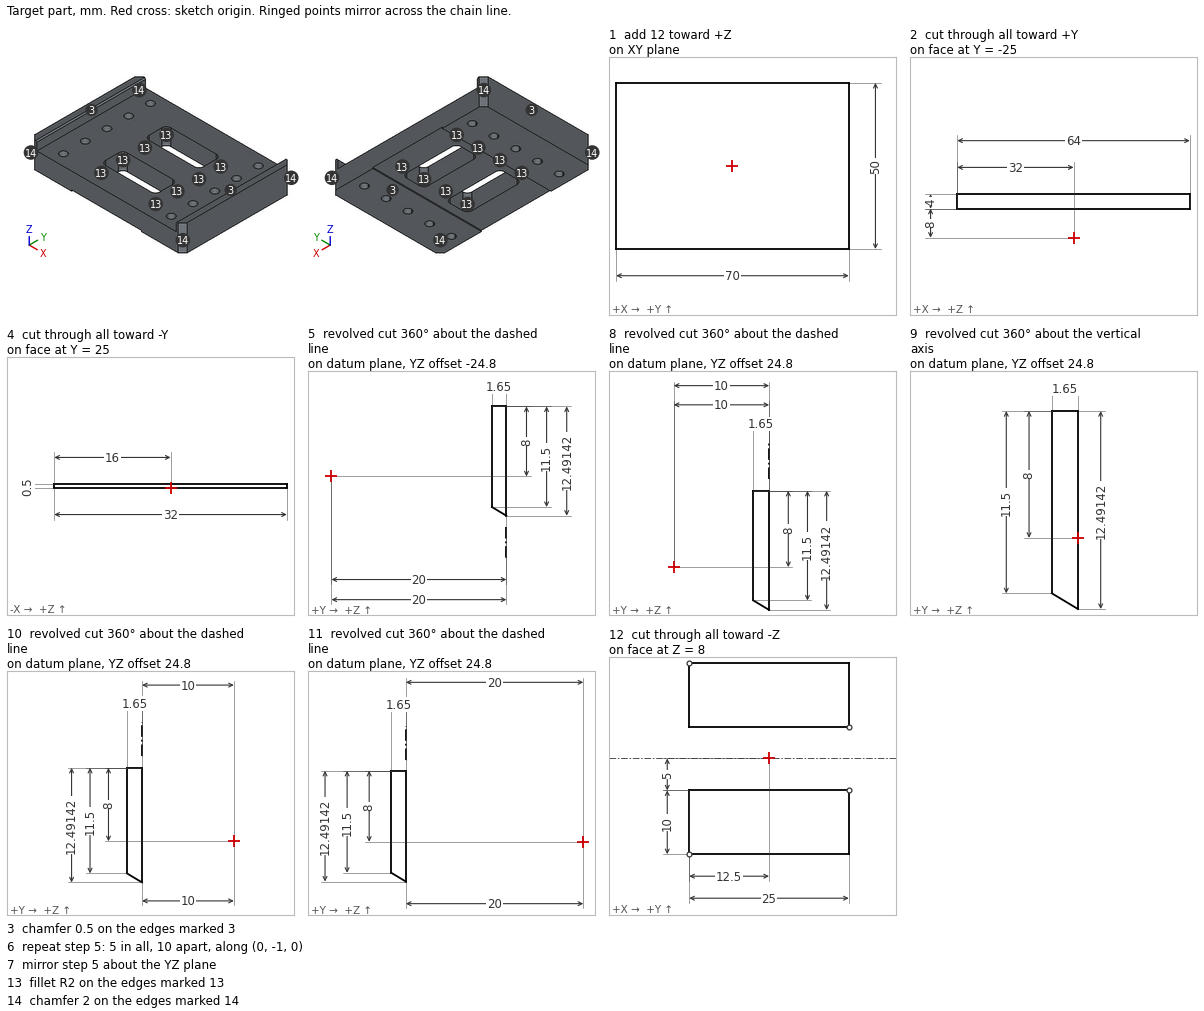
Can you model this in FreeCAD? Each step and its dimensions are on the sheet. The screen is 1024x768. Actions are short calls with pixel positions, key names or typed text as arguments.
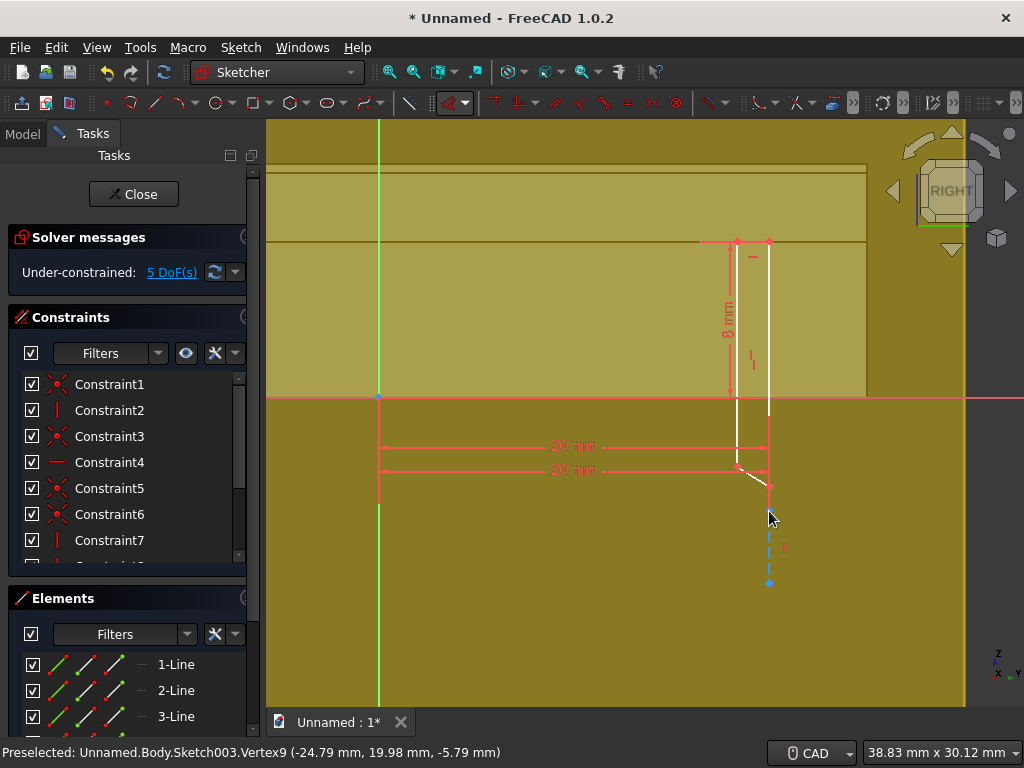
scroll(760, 242, up, 2)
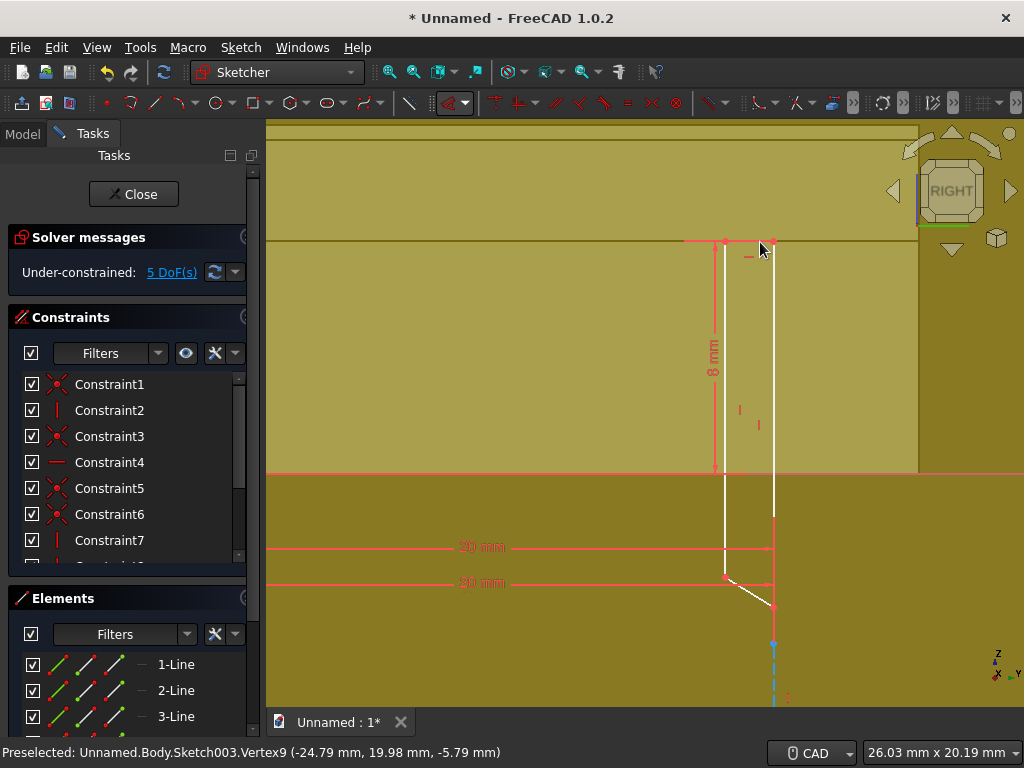
click(759, 241)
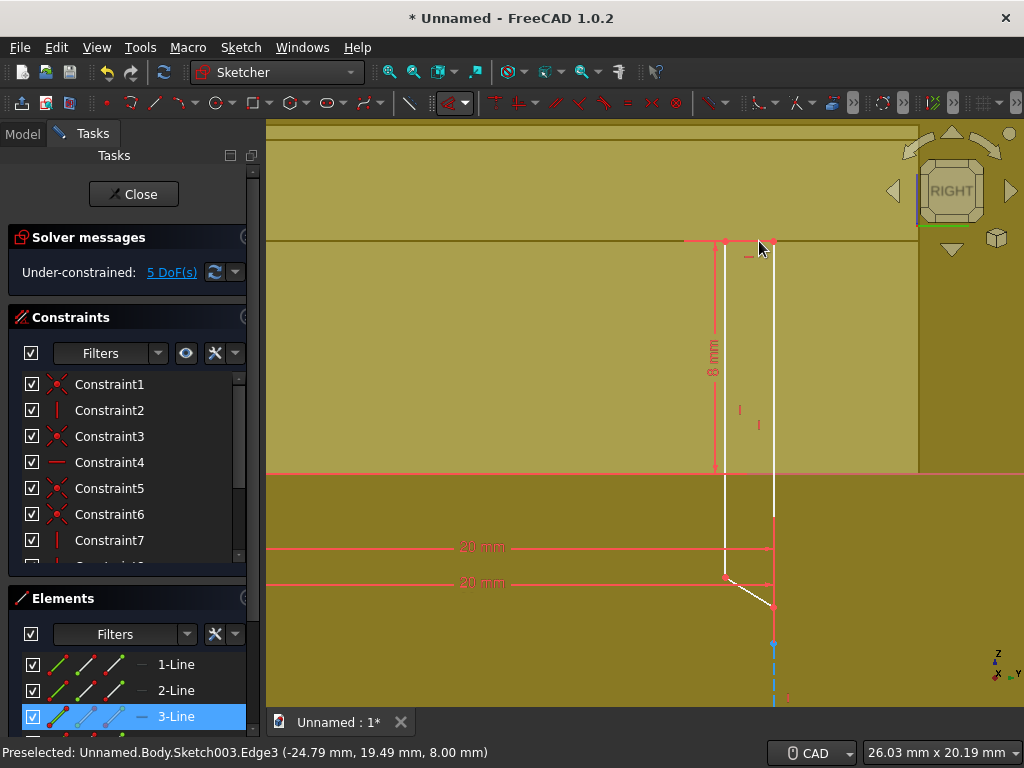
key(l)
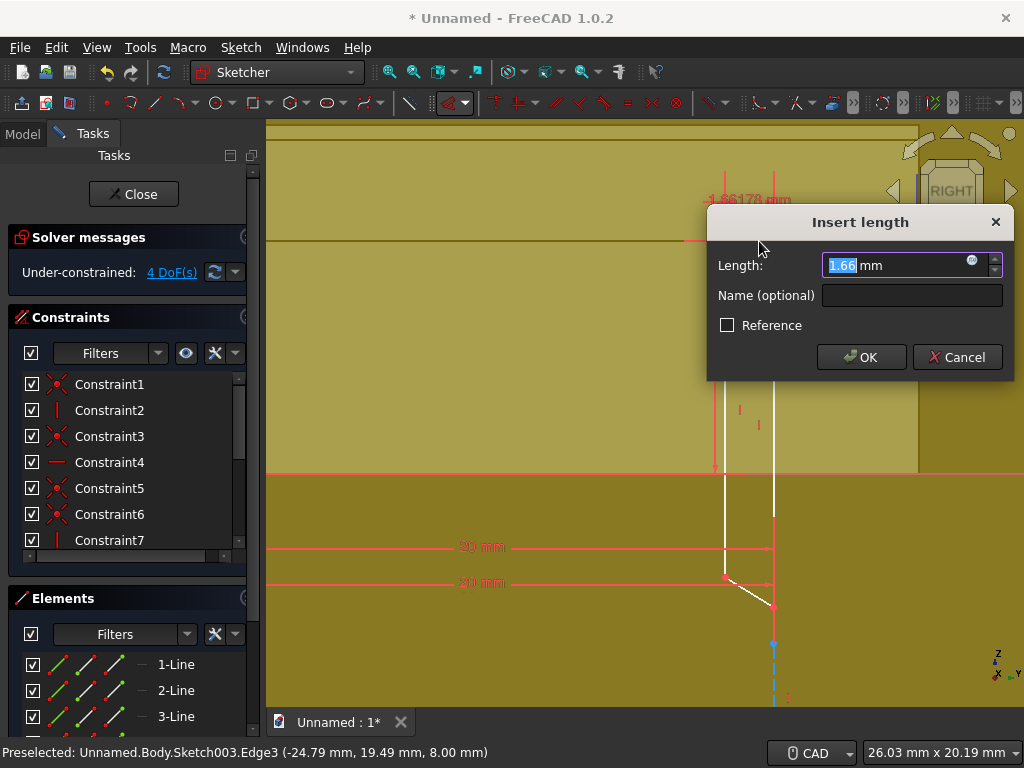
text(1.65)
key(Return)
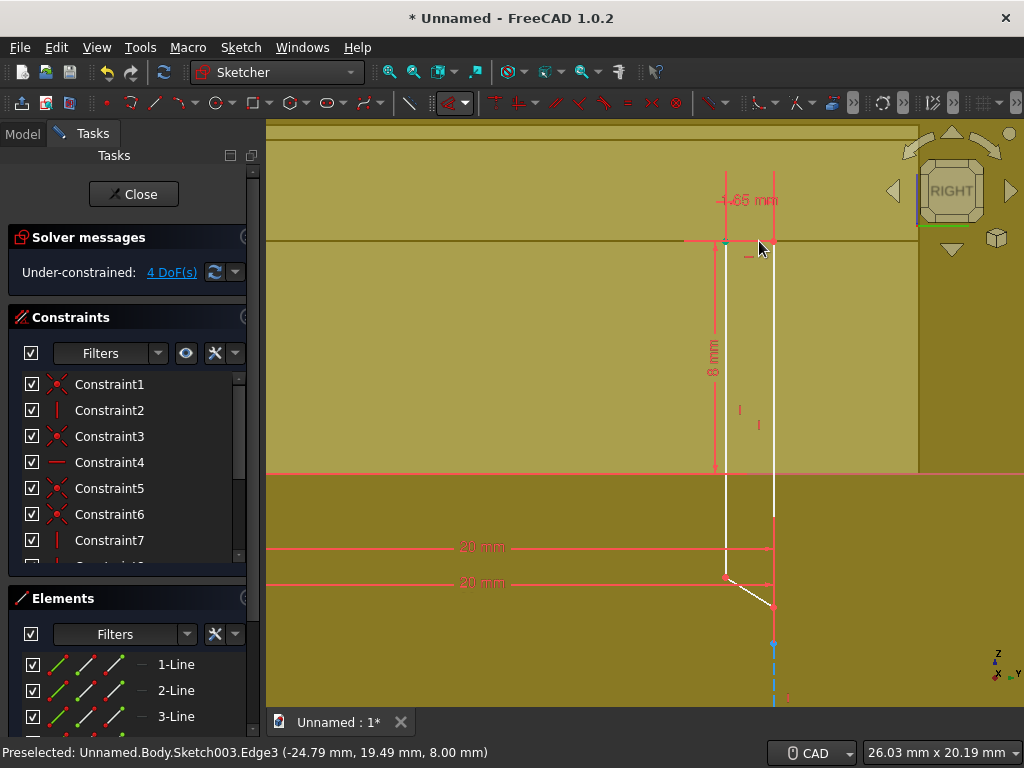
click(726, 342)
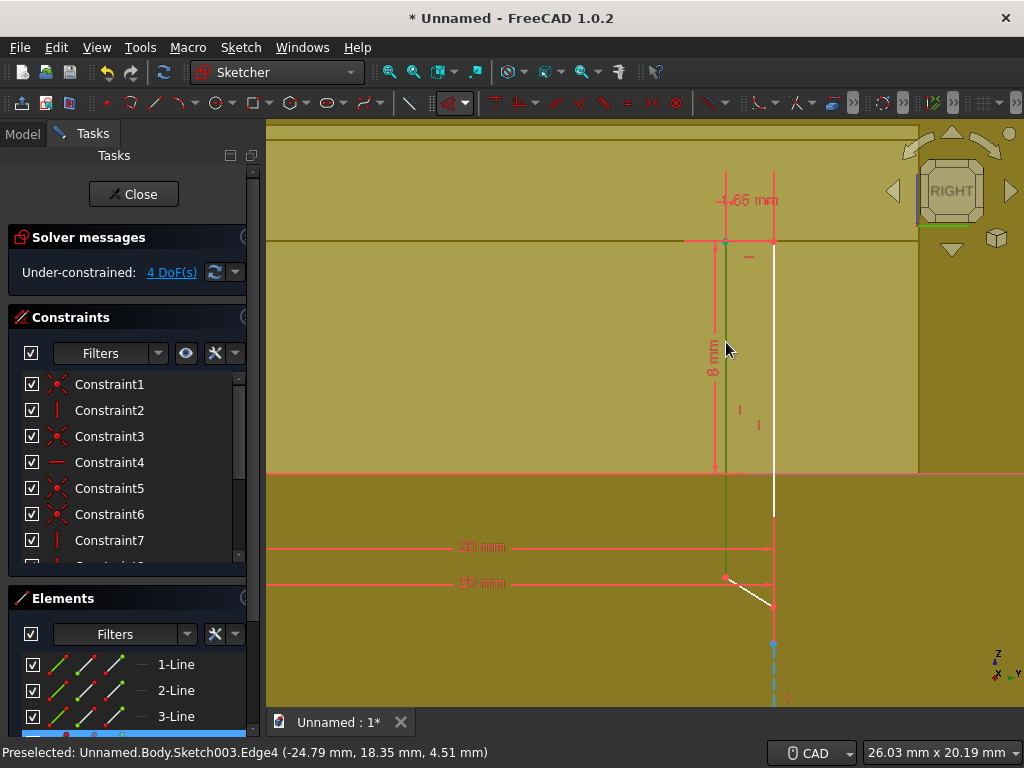
key(i)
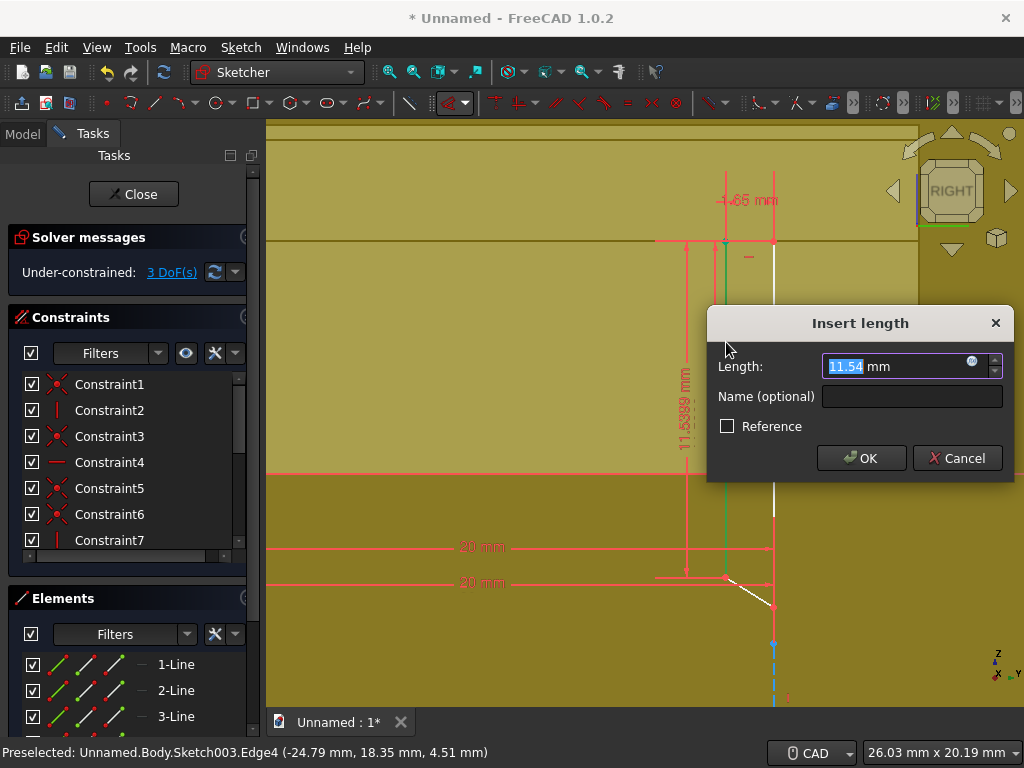
text(11.5)
key(Return)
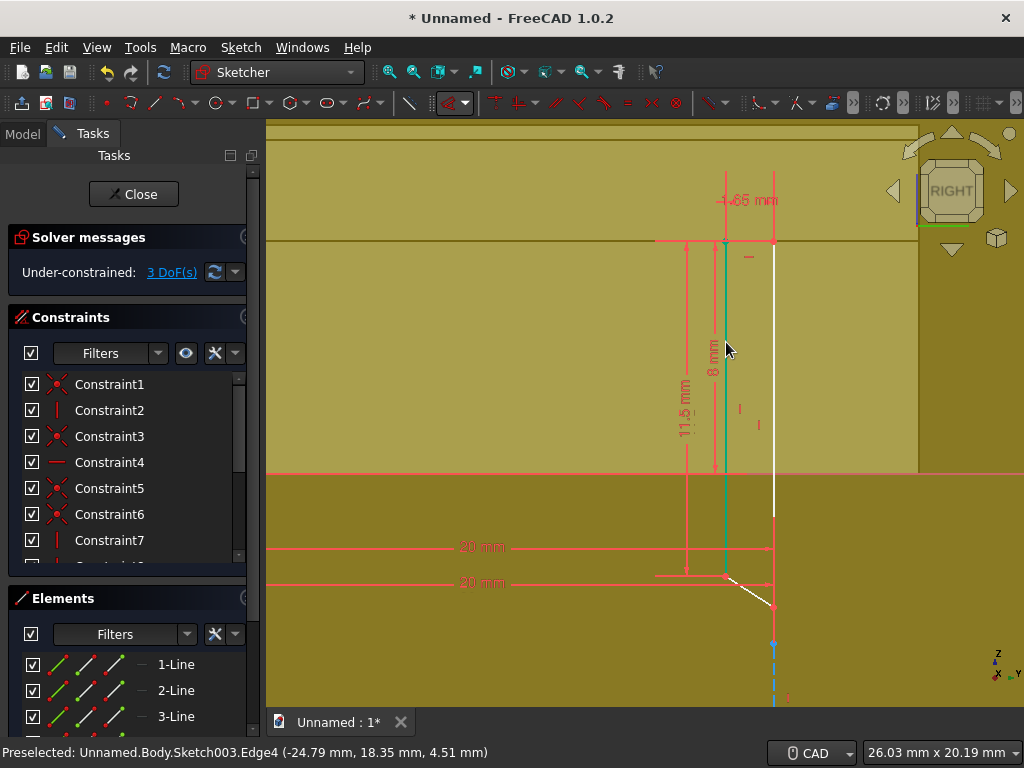
click(774, 498)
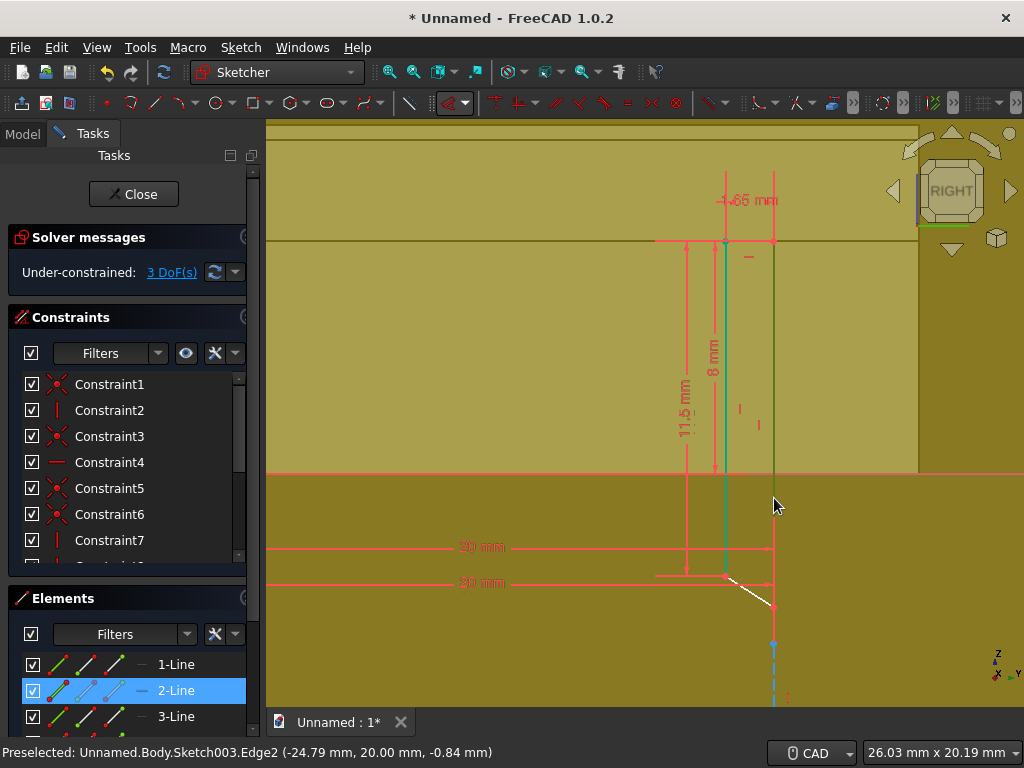
key(i)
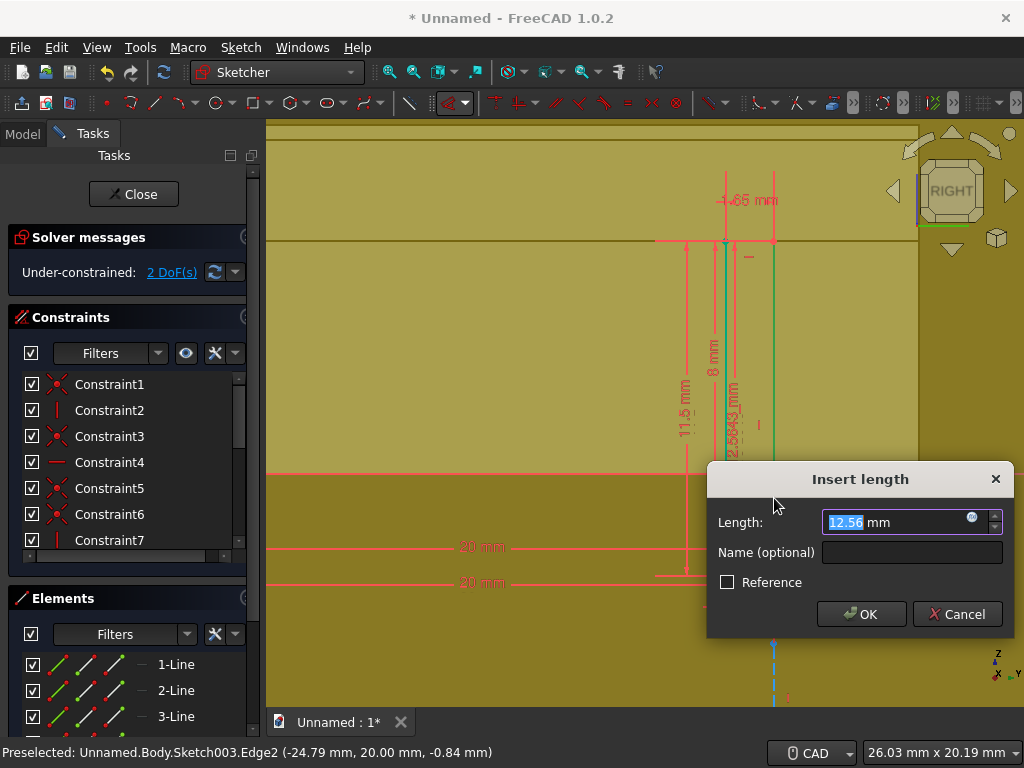
text(12.49142)
key(Return)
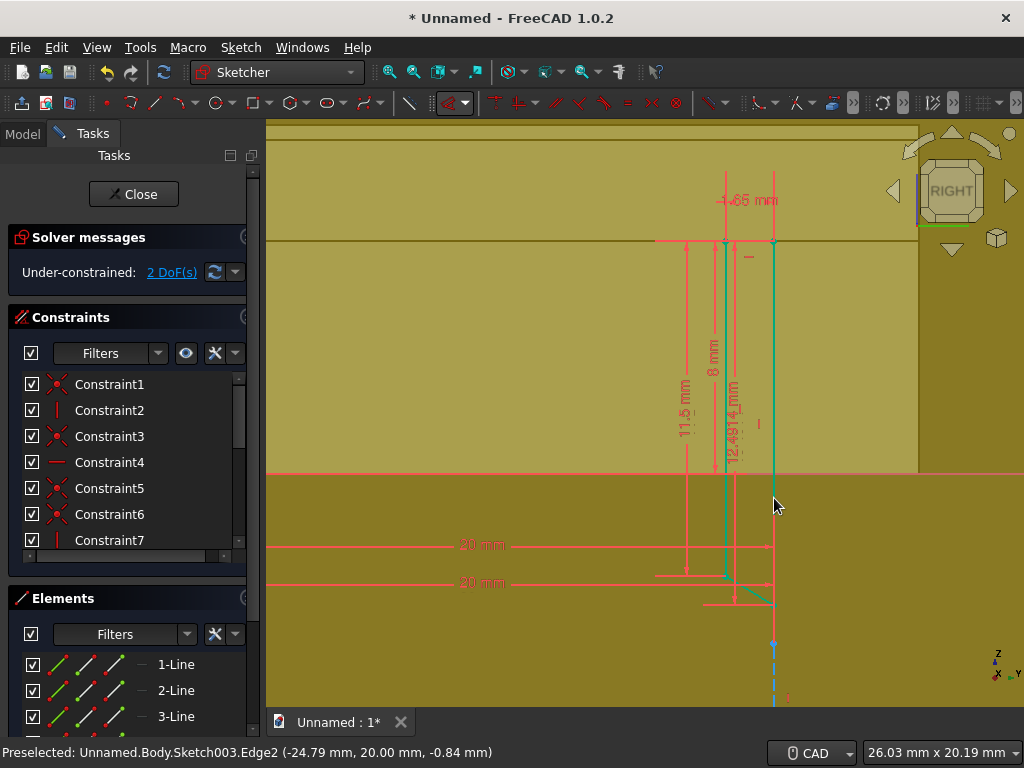
click(134, 194)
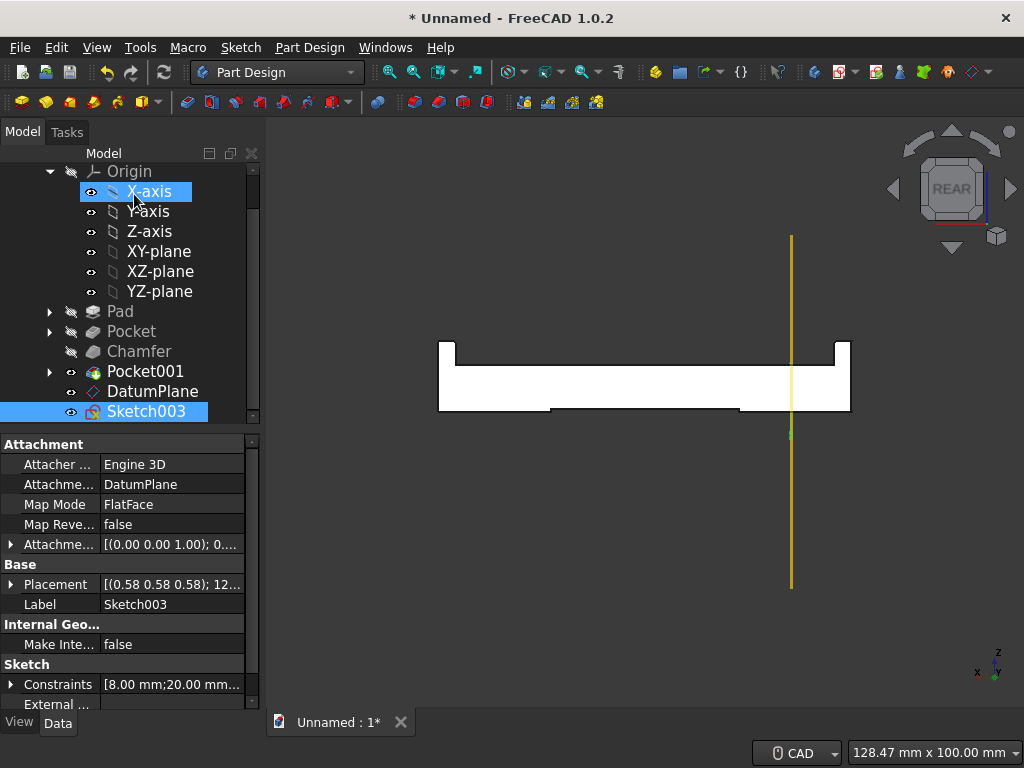
click(236, 102)